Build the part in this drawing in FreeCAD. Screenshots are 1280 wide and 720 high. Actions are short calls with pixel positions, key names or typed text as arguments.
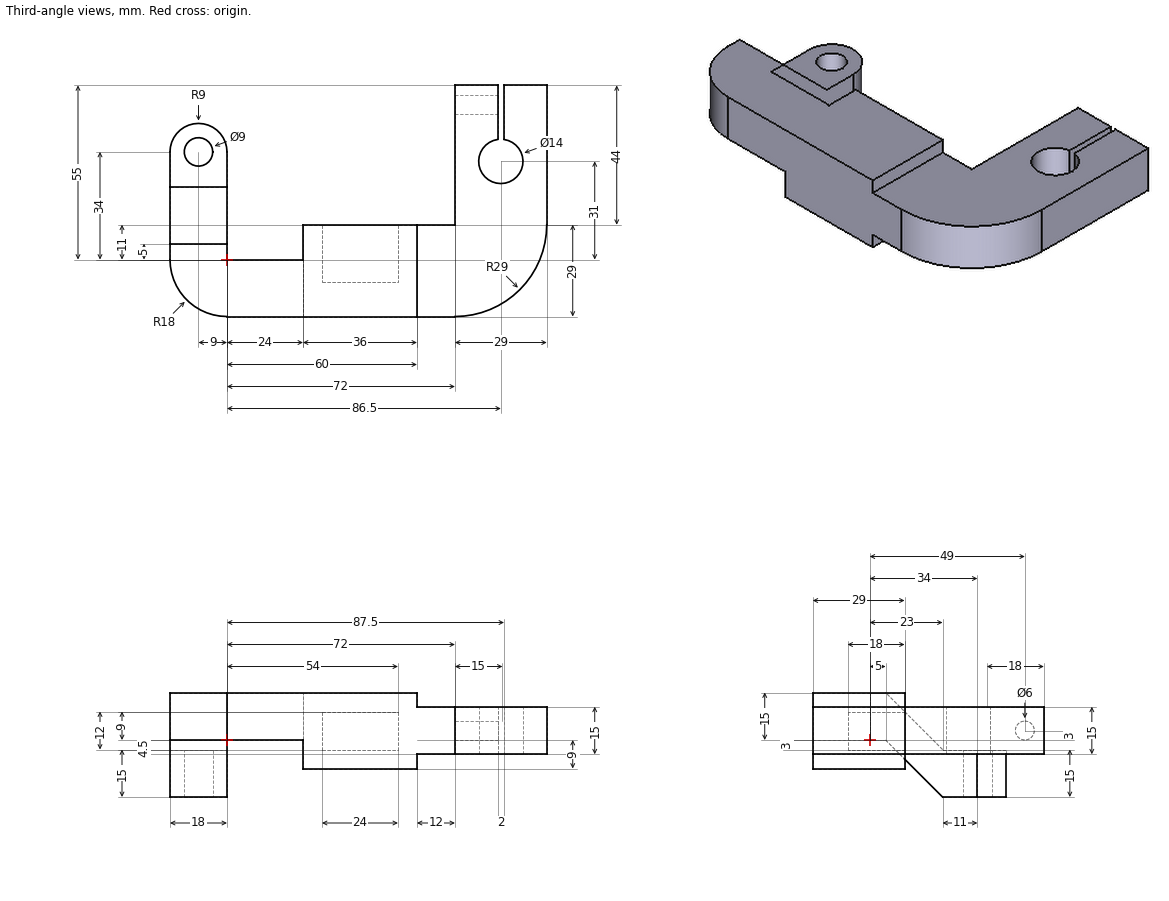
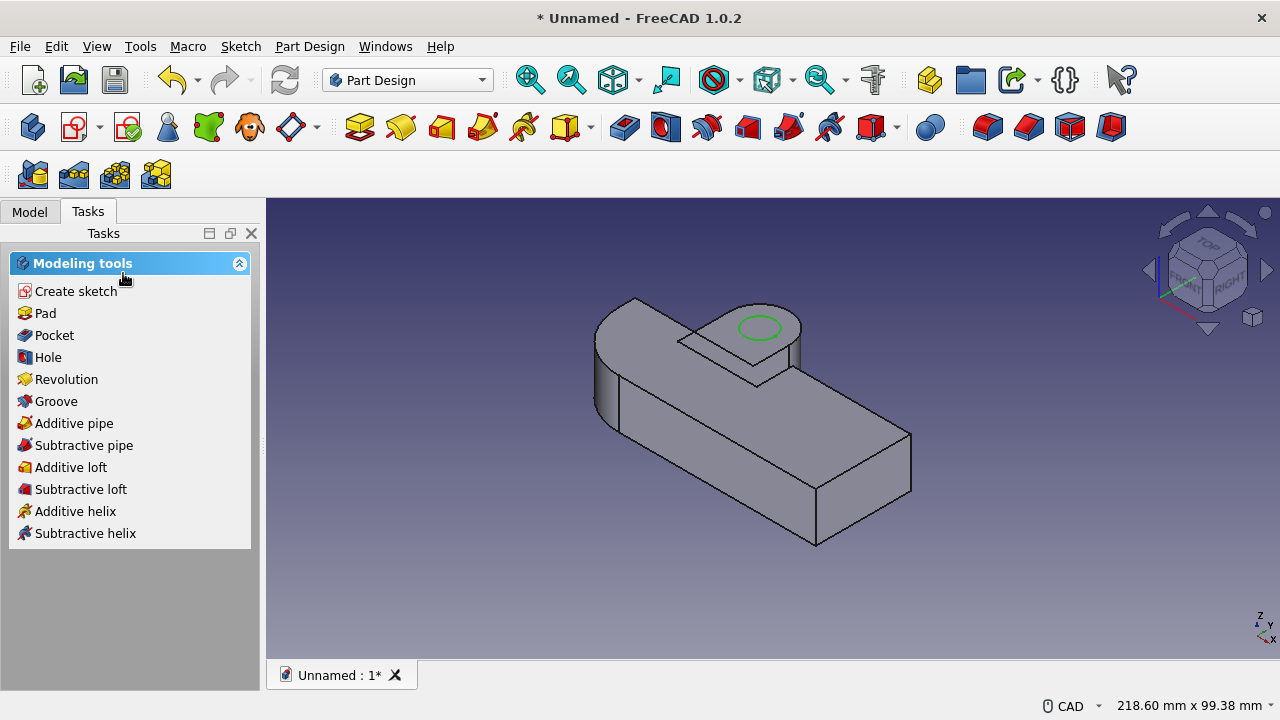
click(625, 128)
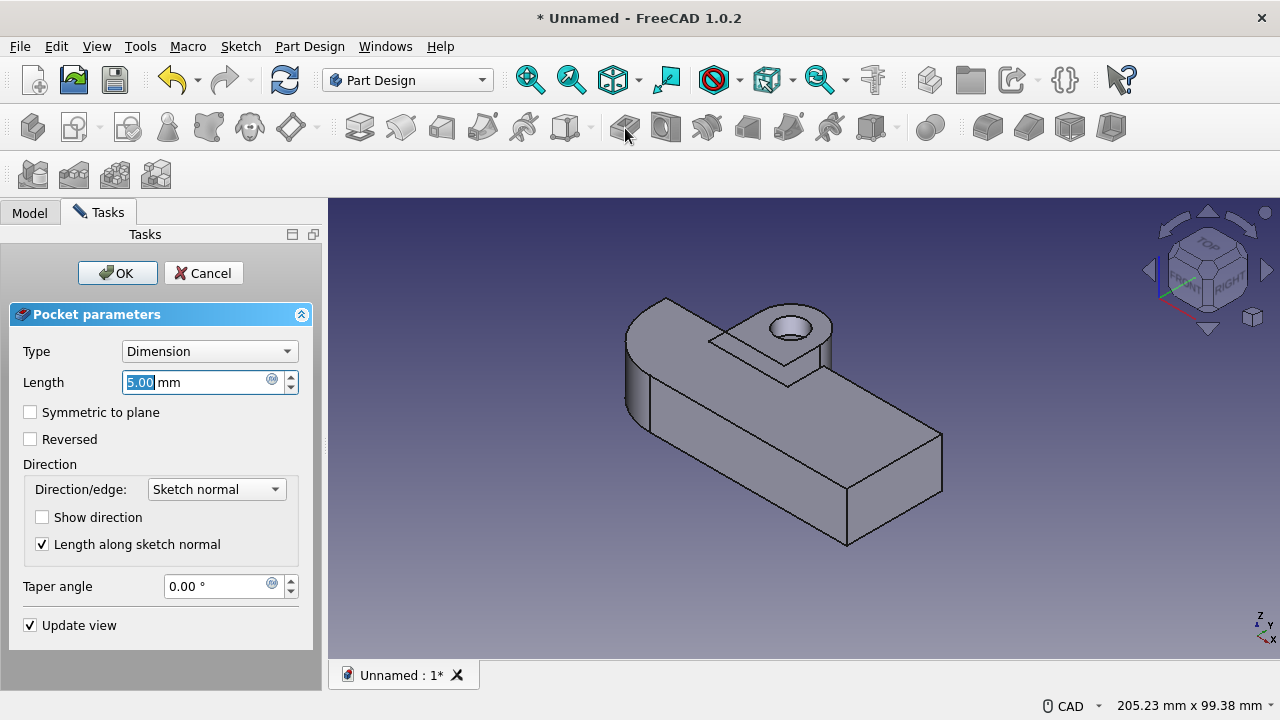
text(15)
key(Tab)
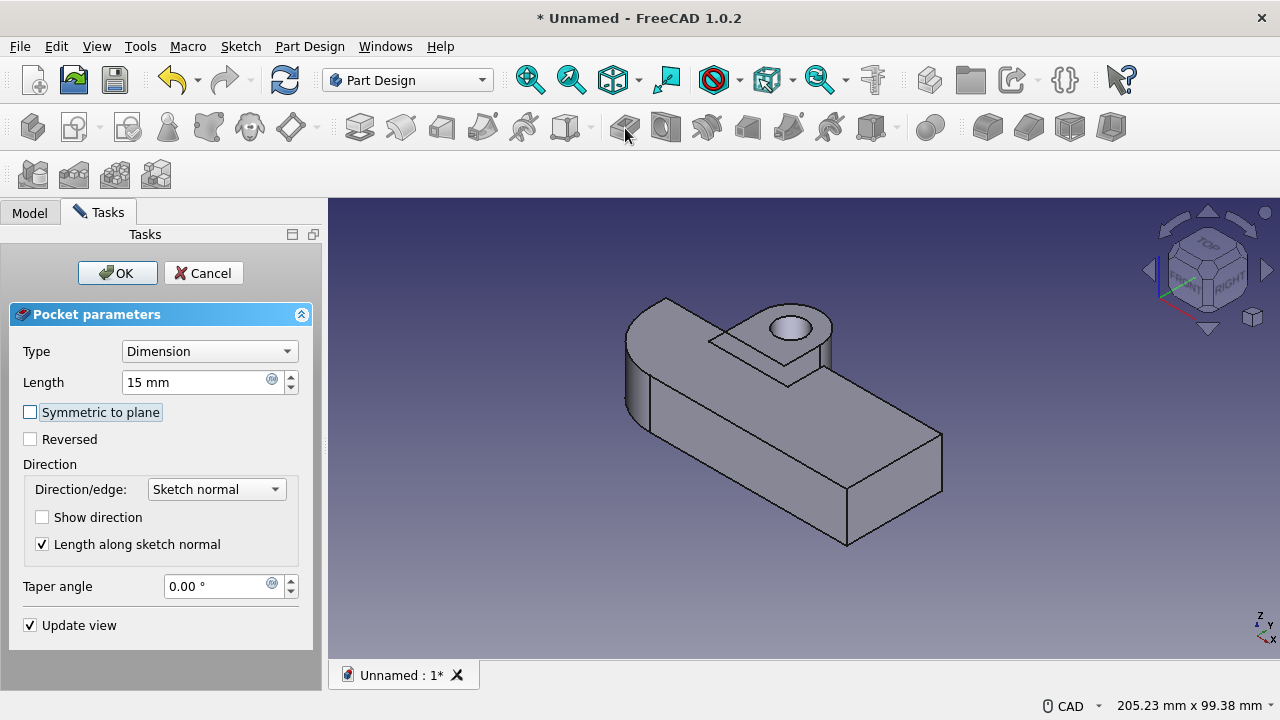
click(118, 273)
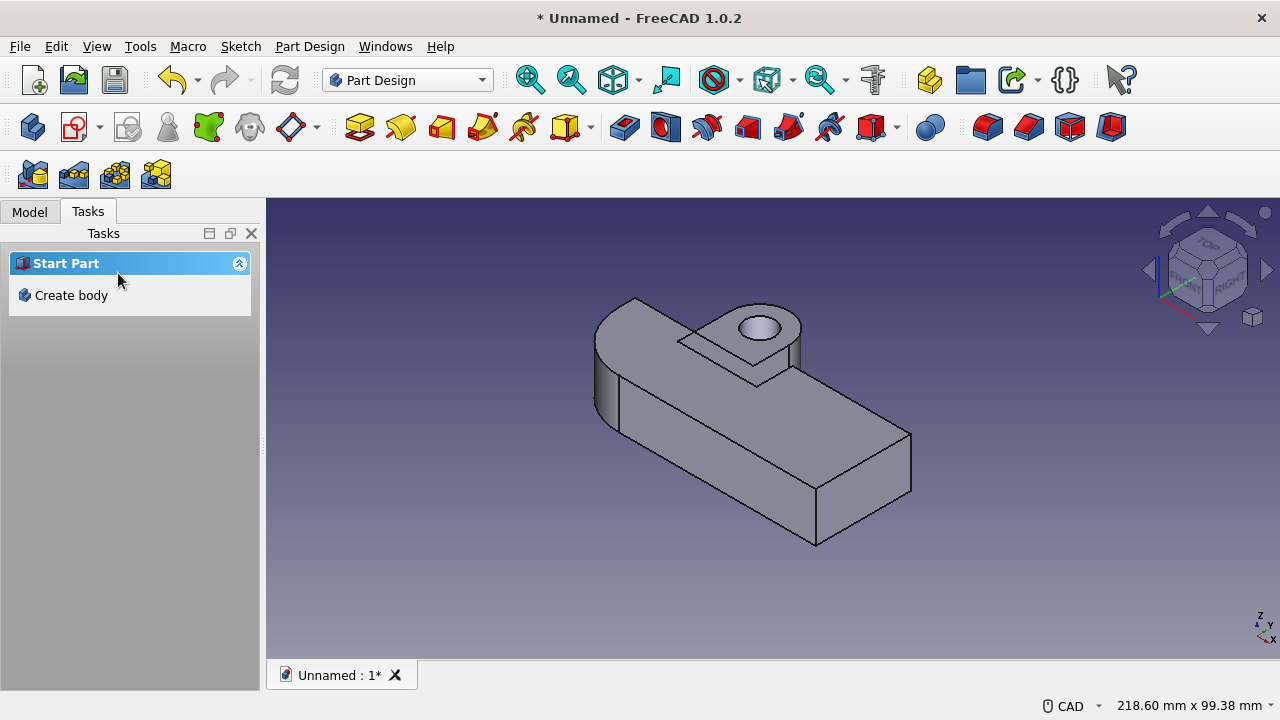
click(74, 128)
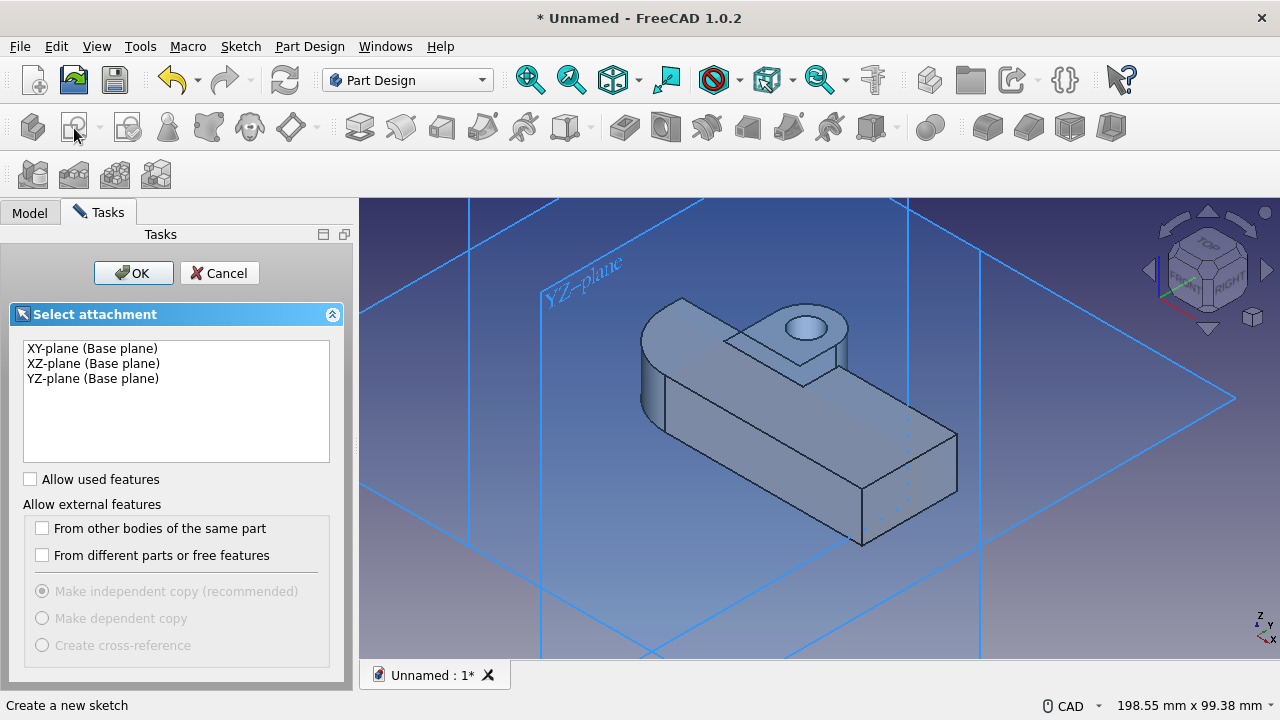
click(84, 348)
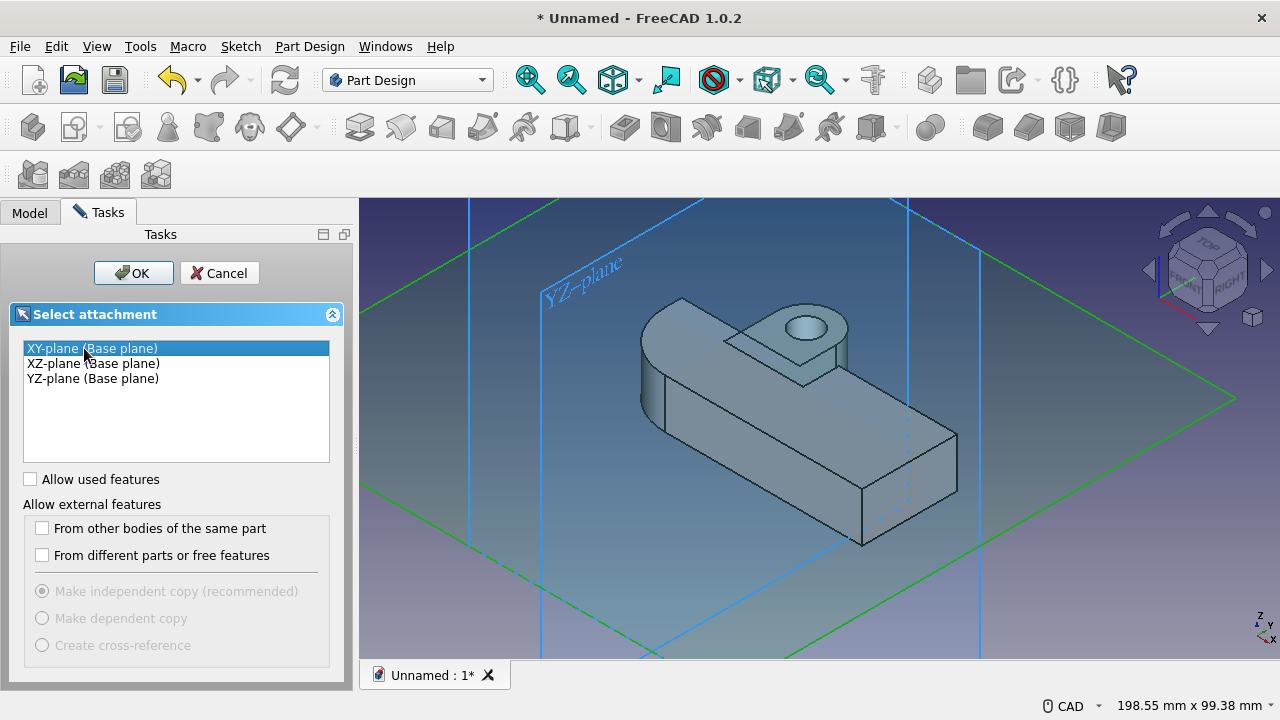
click(134, 273)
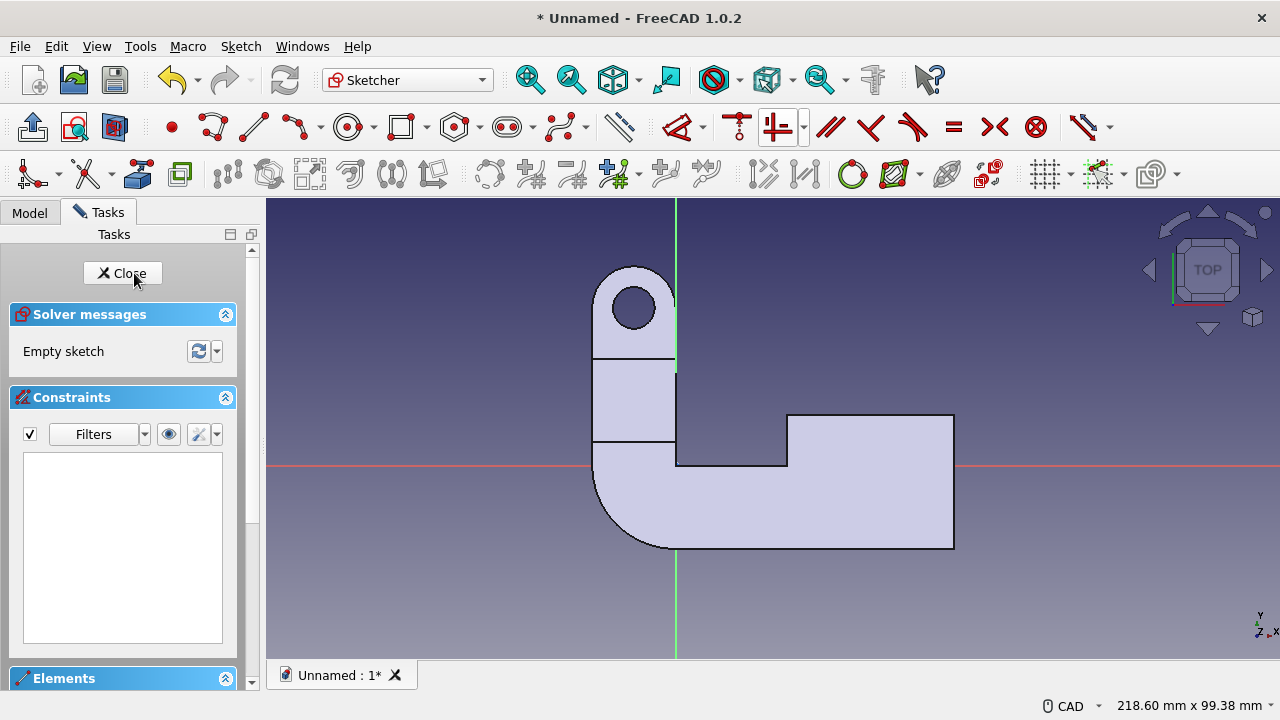
click(115, 128)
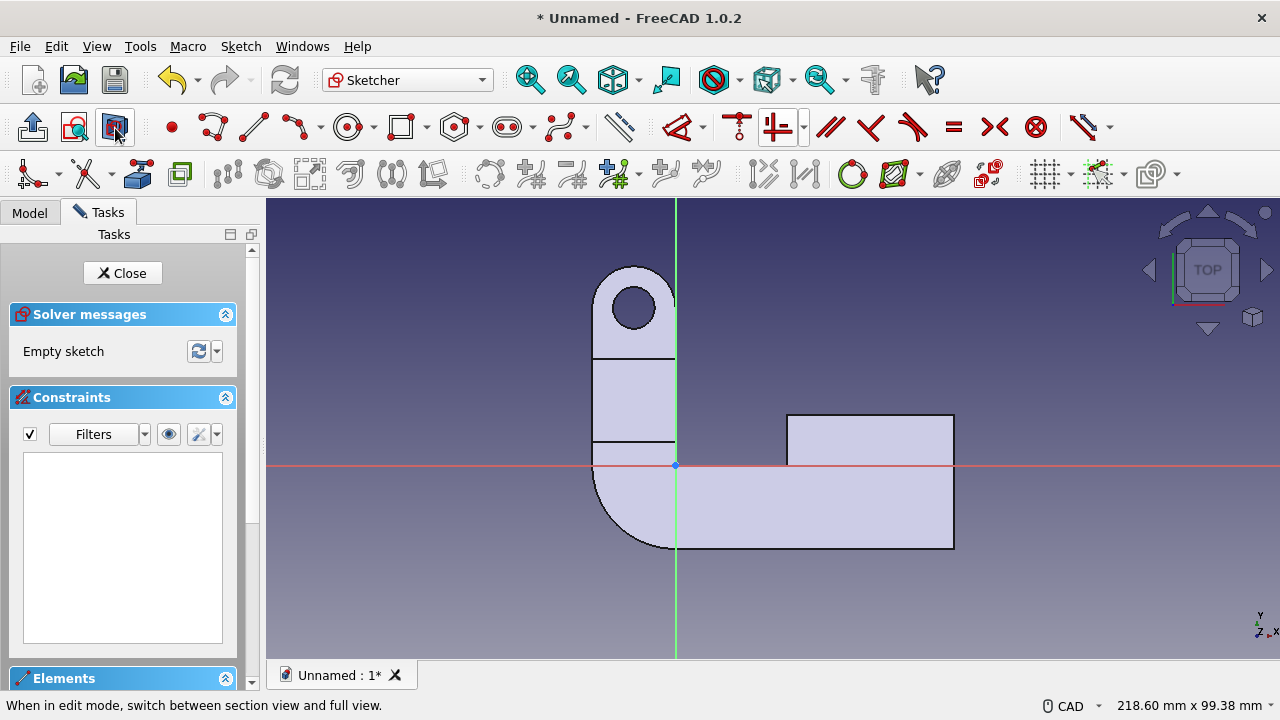
scroll(905, 525, up, 4)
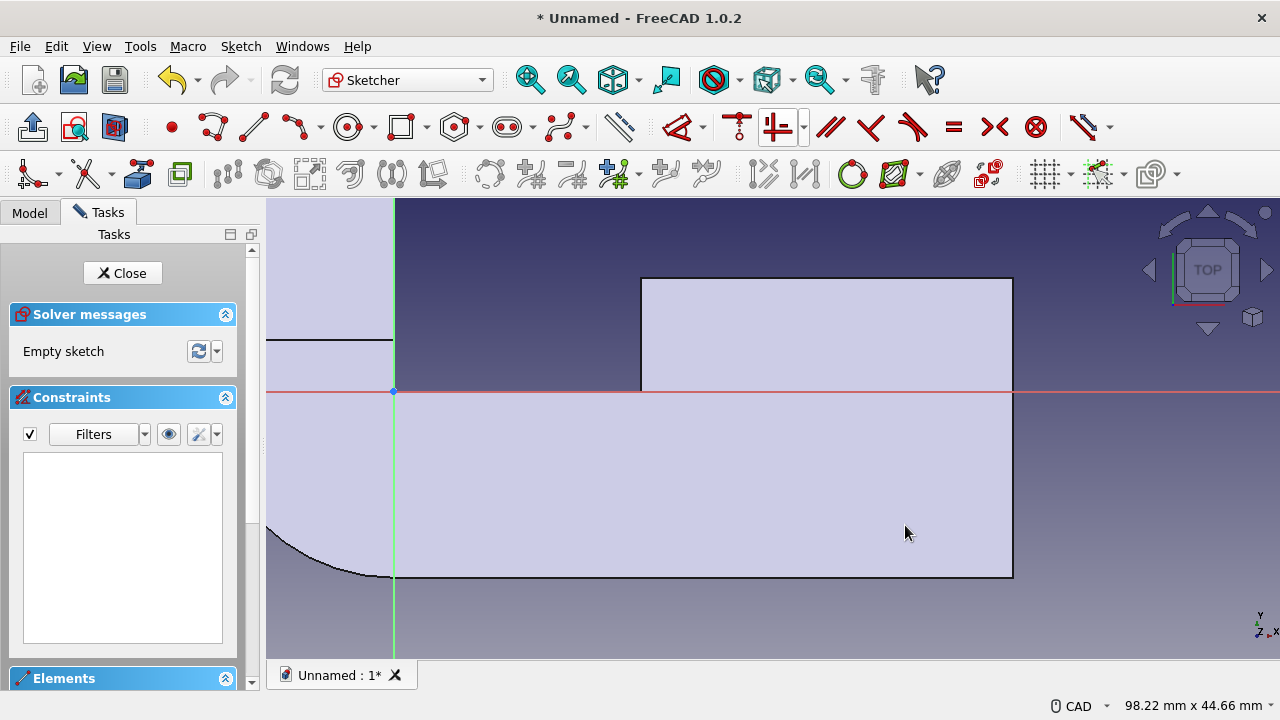
click(400, 128)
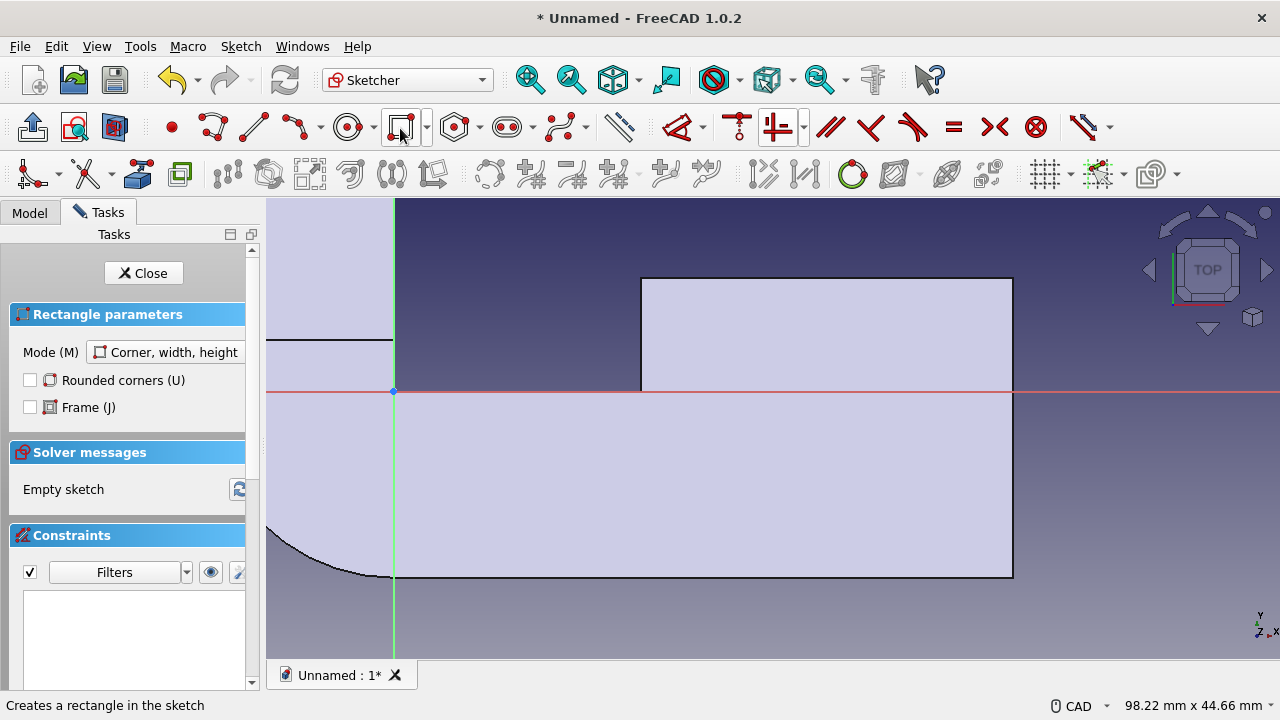
click(641, 278)
move(1013, 578)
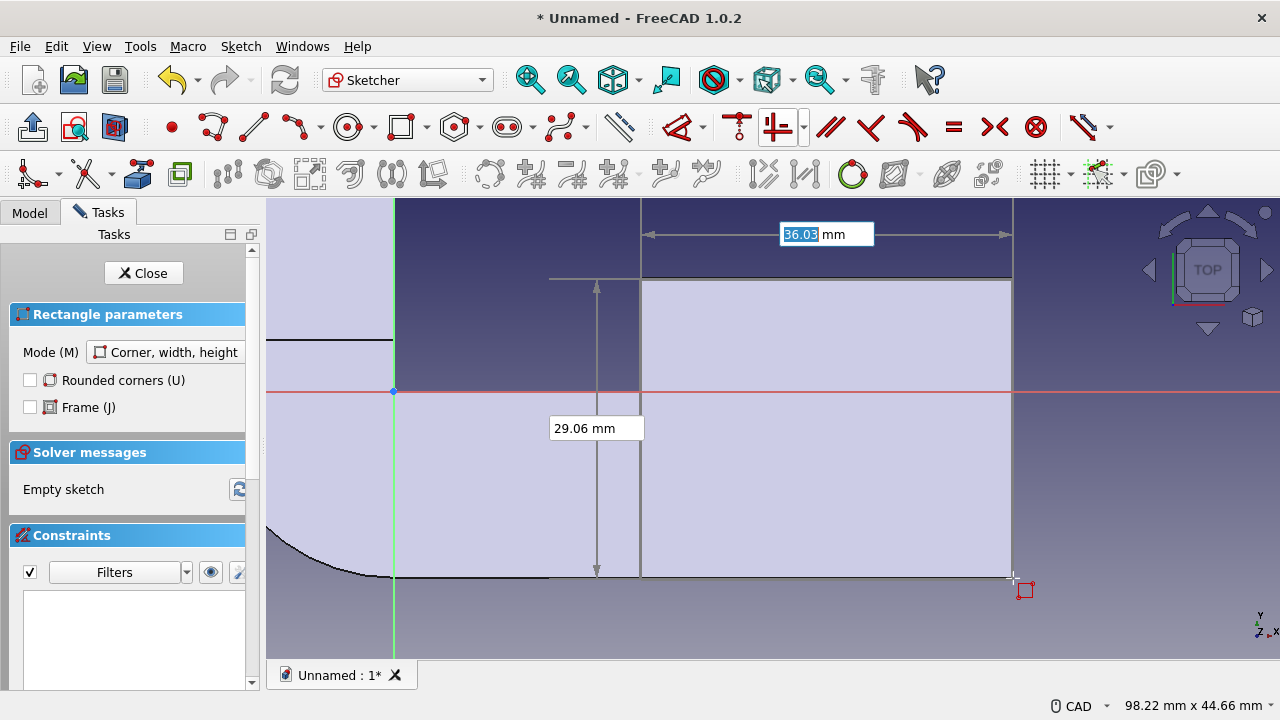
text(36)
key(Tab)
text(29)
key(Return)
key(Escape)